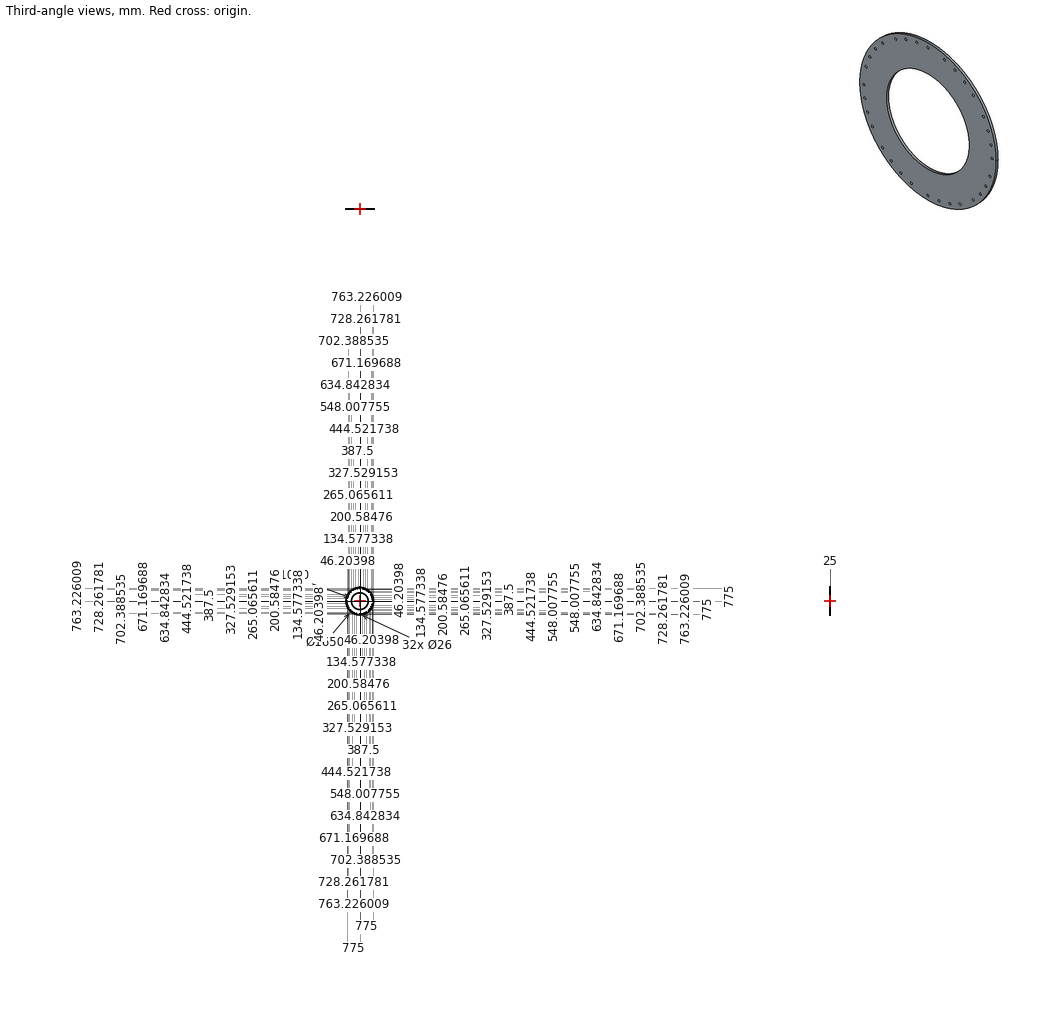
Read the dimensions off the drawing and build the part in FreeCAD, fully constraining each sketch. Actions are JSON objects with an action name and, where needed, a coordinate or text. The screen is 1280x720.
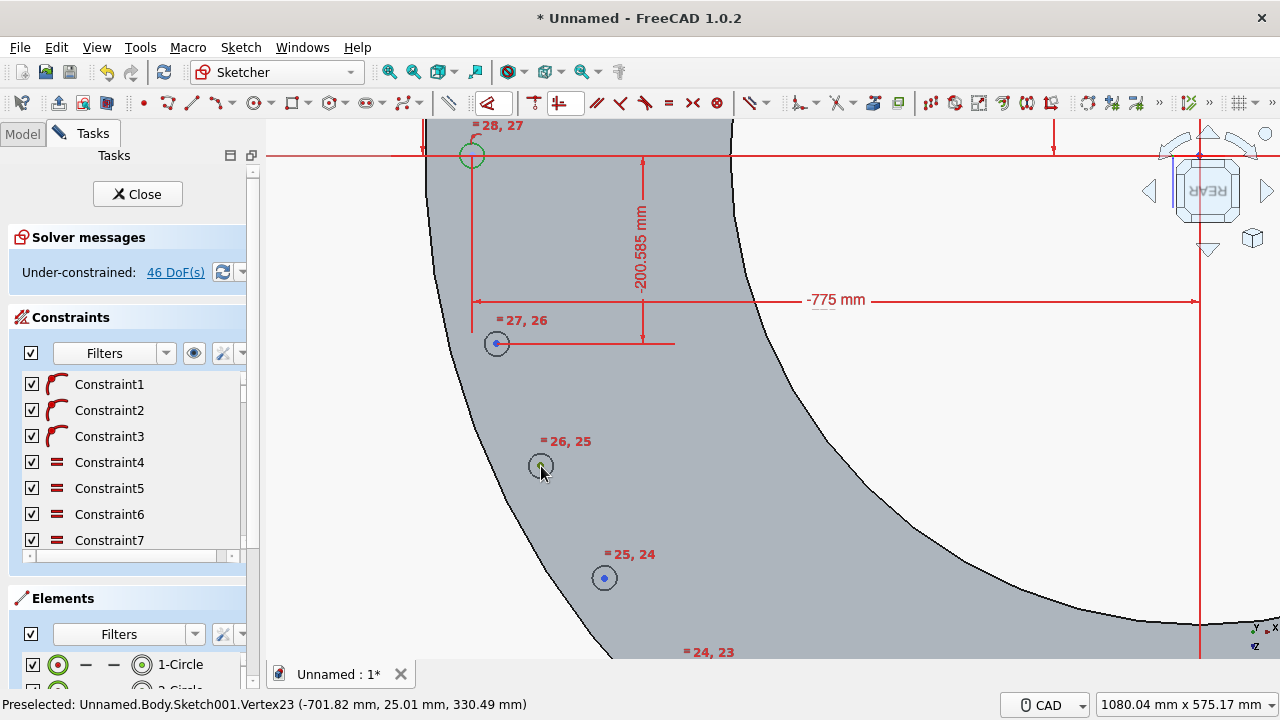
{"action": "left_click", "coordinate": [497, 344]}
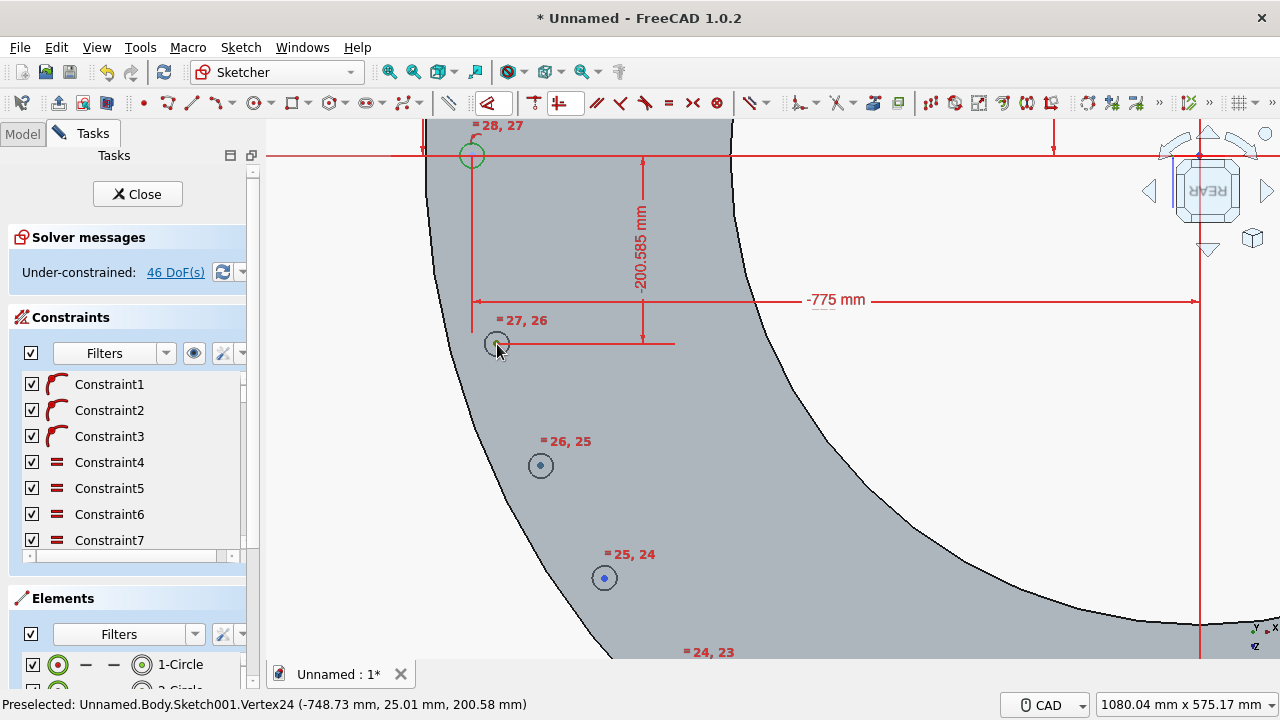
{"action": "key", "text": "l"}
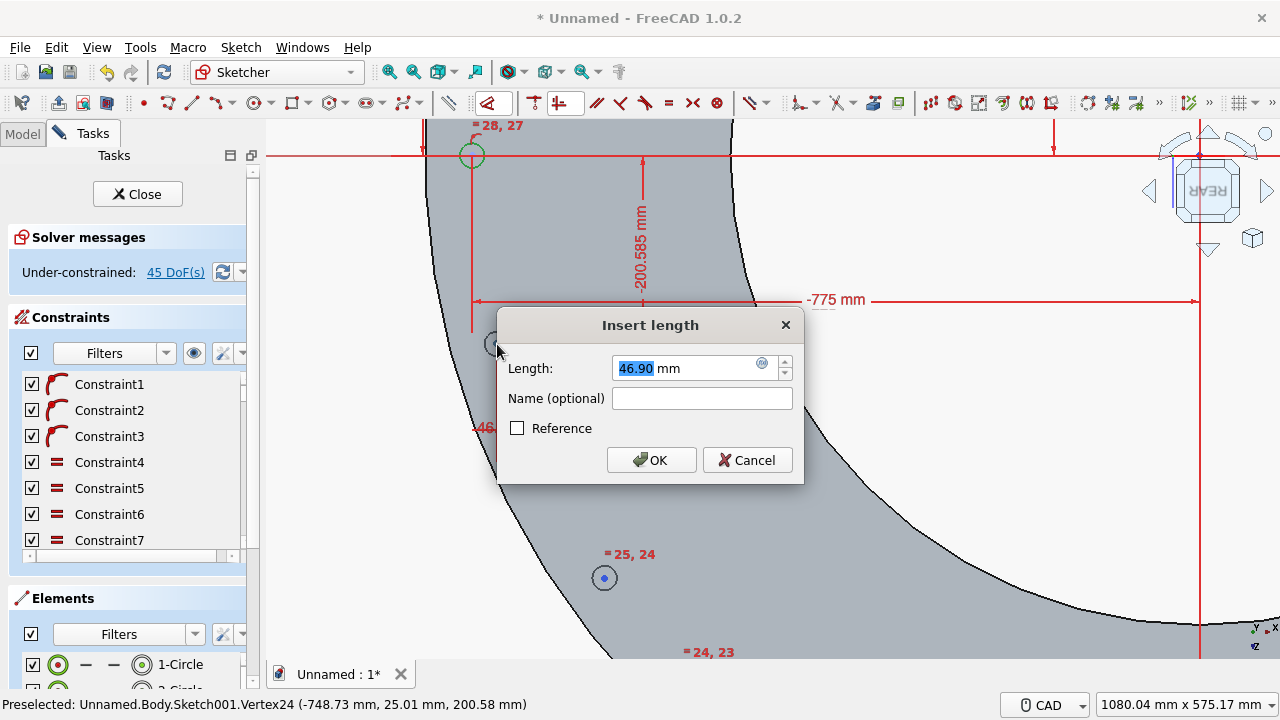
{"action": "type", "text": "46.20398"}
{"action": "key", "text": "Return"}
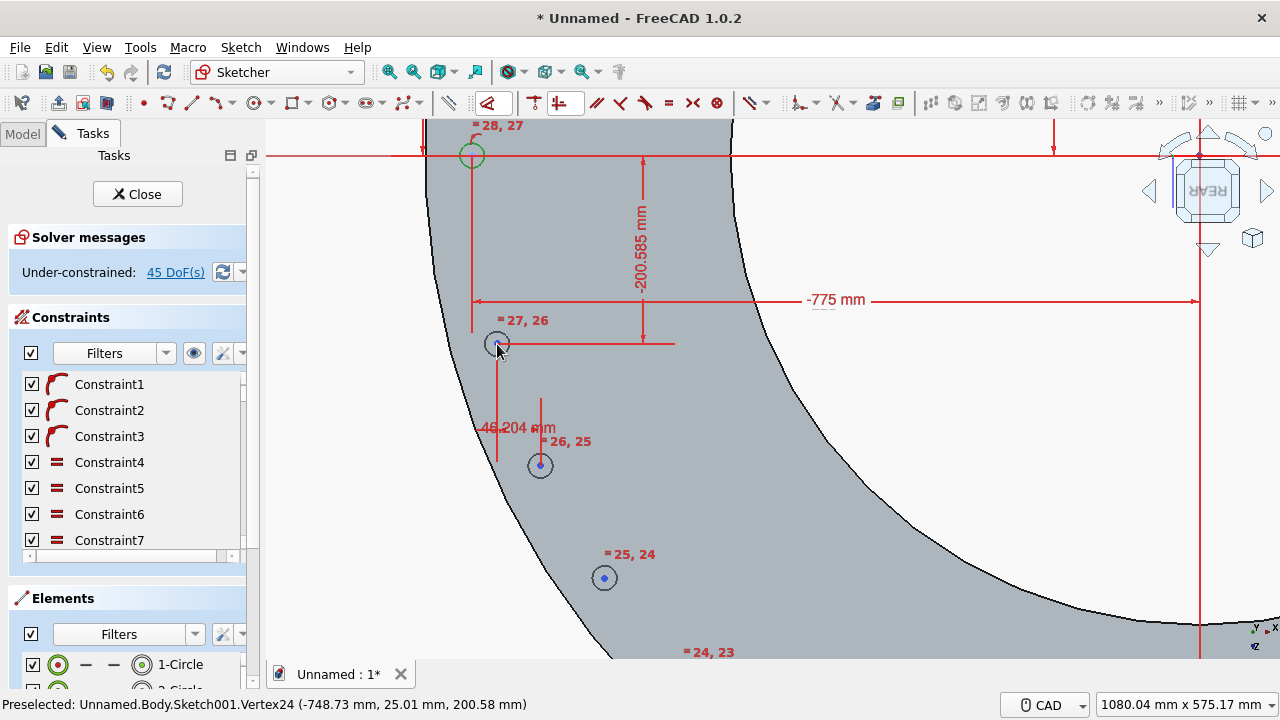
{"action": "scroll", "coordinate": [542, 465], "scroll_direction": "down", "scroll_amount": 7}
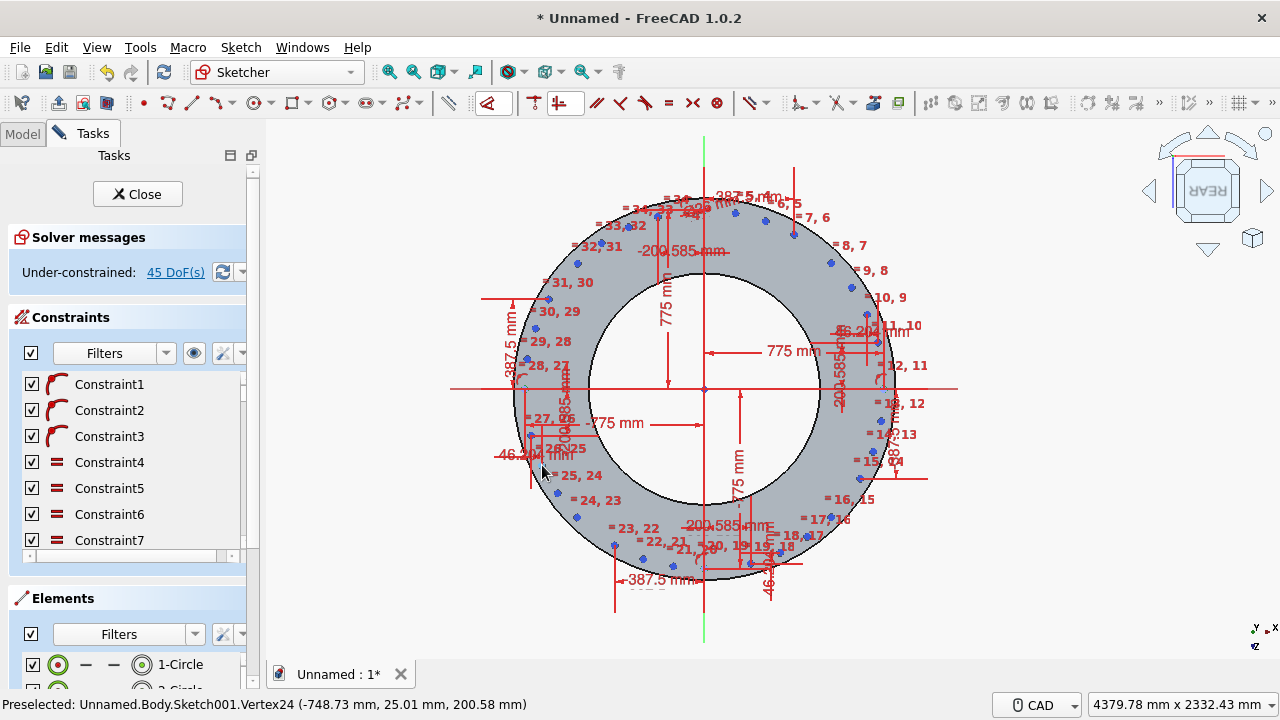
{"action": "scroll", "coordinate": [629, 227], "scroll_direction": "up", "scroll_amount": 7}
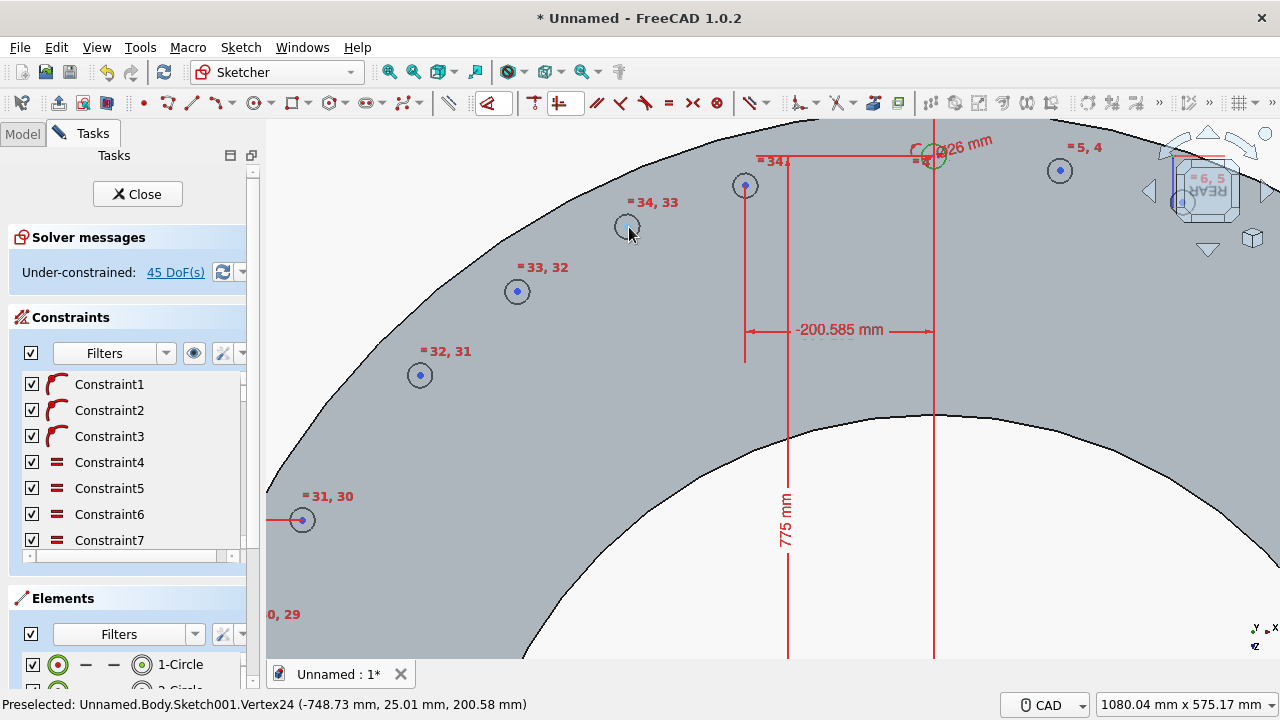
{"action": "left_click", "coordinate": [627, 227]}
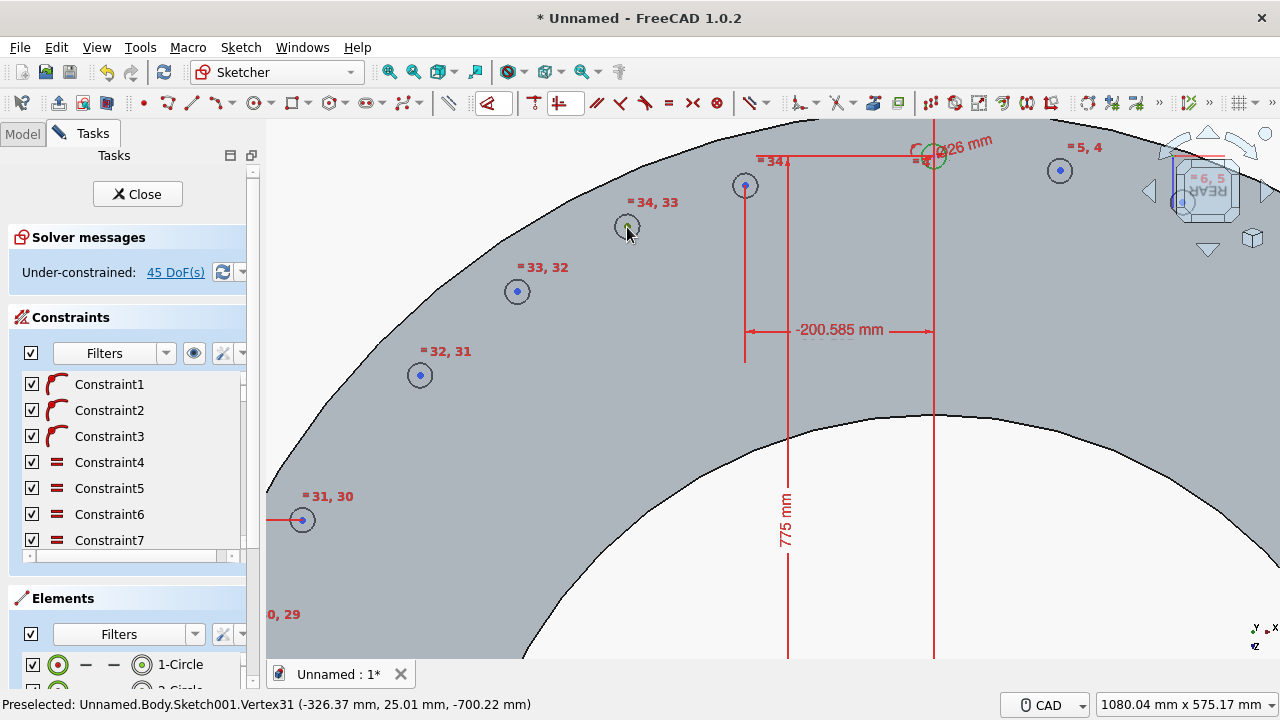
{"action": "left_click", "coordinate": [745, 186]}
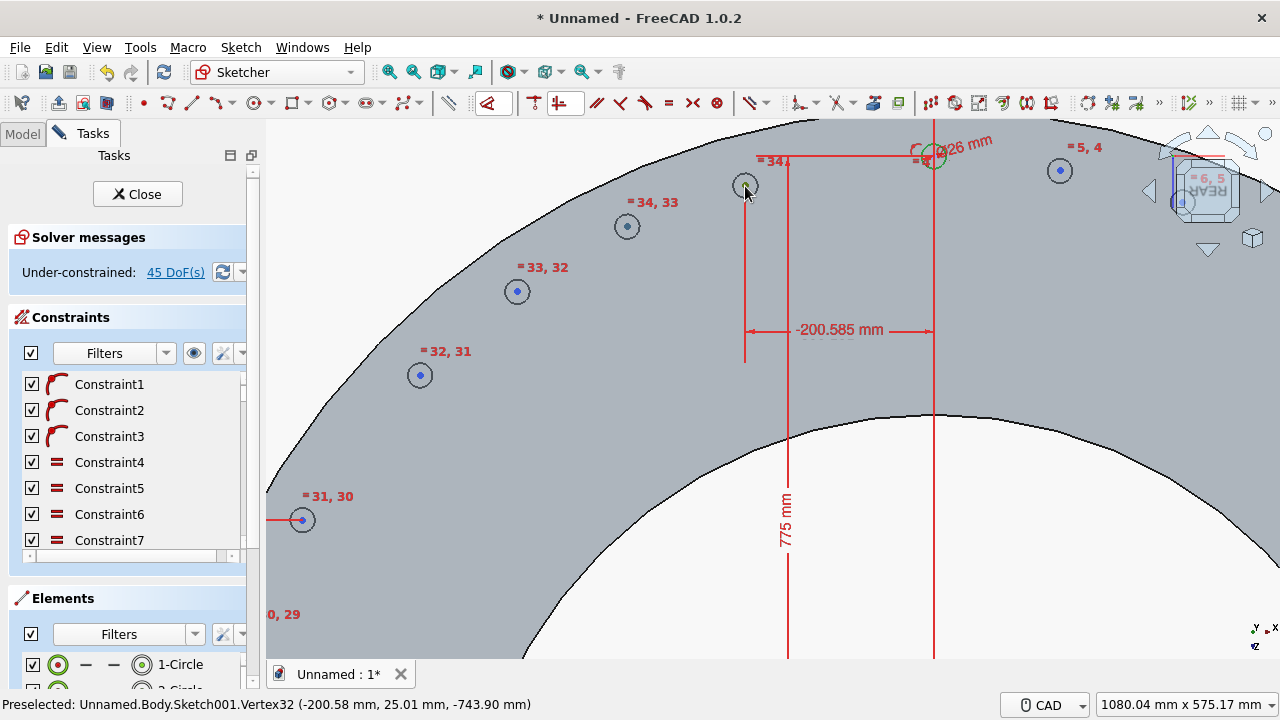
{"action": "key", "text": "i"}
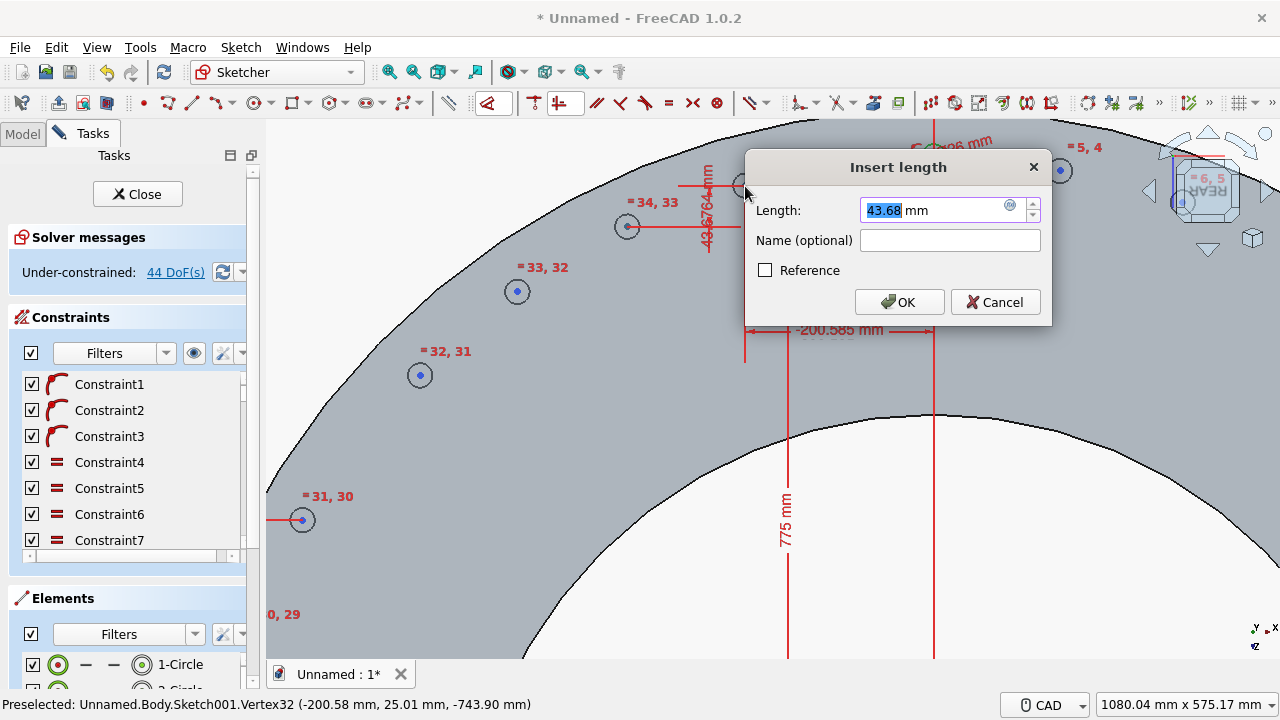
{"action": "type", "text": "46.20398"}
{"action": "key", "text": "Return"}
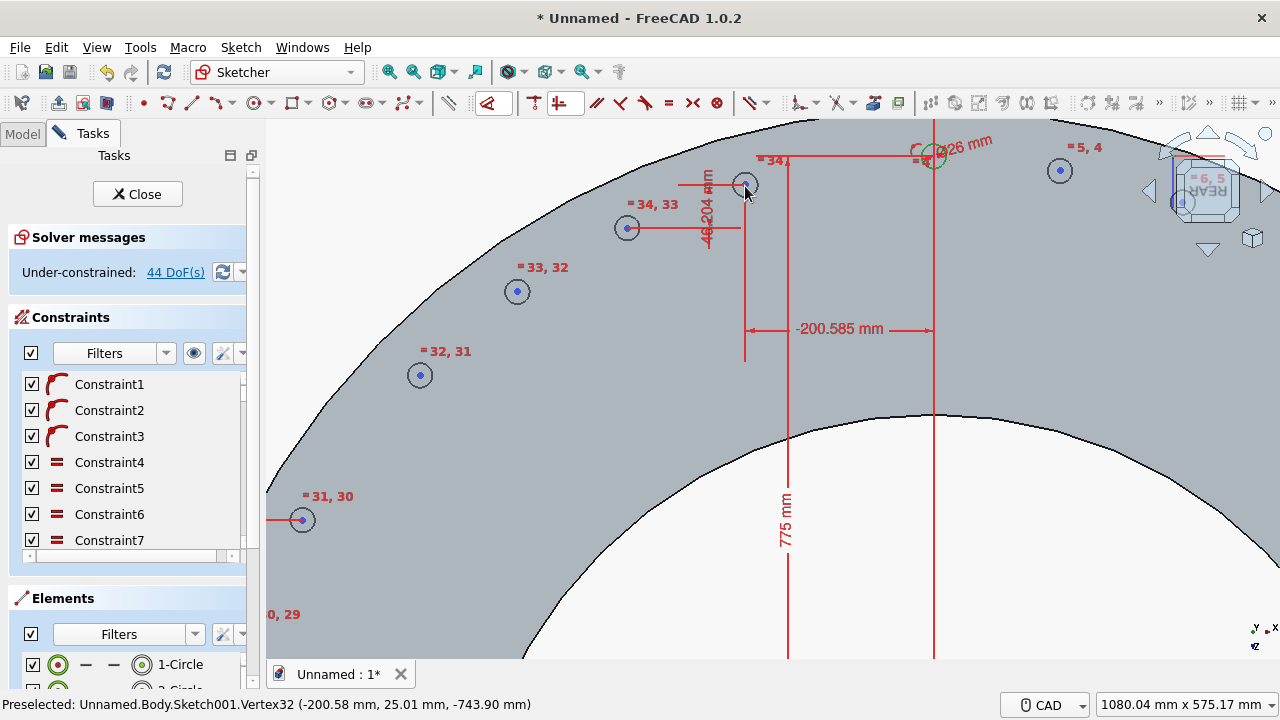
{"action": "scroll", "coordinate": [629, 227], "scroll_direction": "down", "scroll_amount": 7}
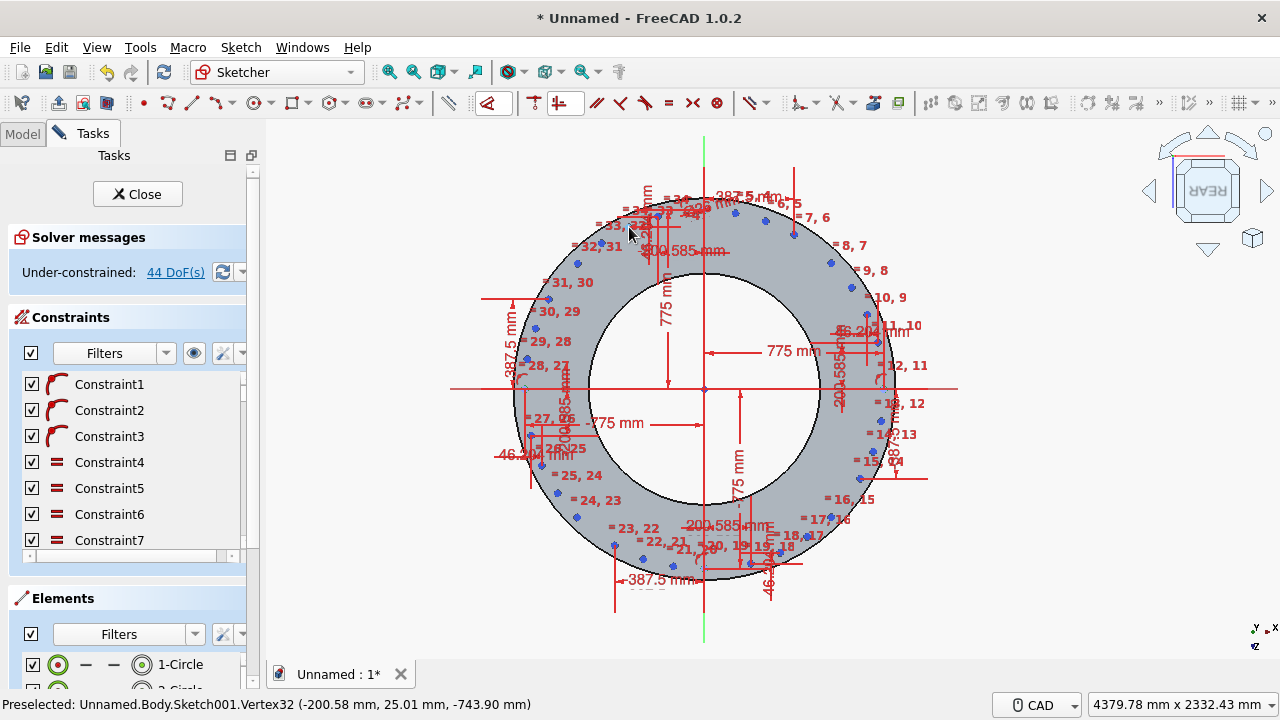
{"action": "scroll", "coordinate": [736, 213], "scroll_direction": "up", "scroll_amount": 2}